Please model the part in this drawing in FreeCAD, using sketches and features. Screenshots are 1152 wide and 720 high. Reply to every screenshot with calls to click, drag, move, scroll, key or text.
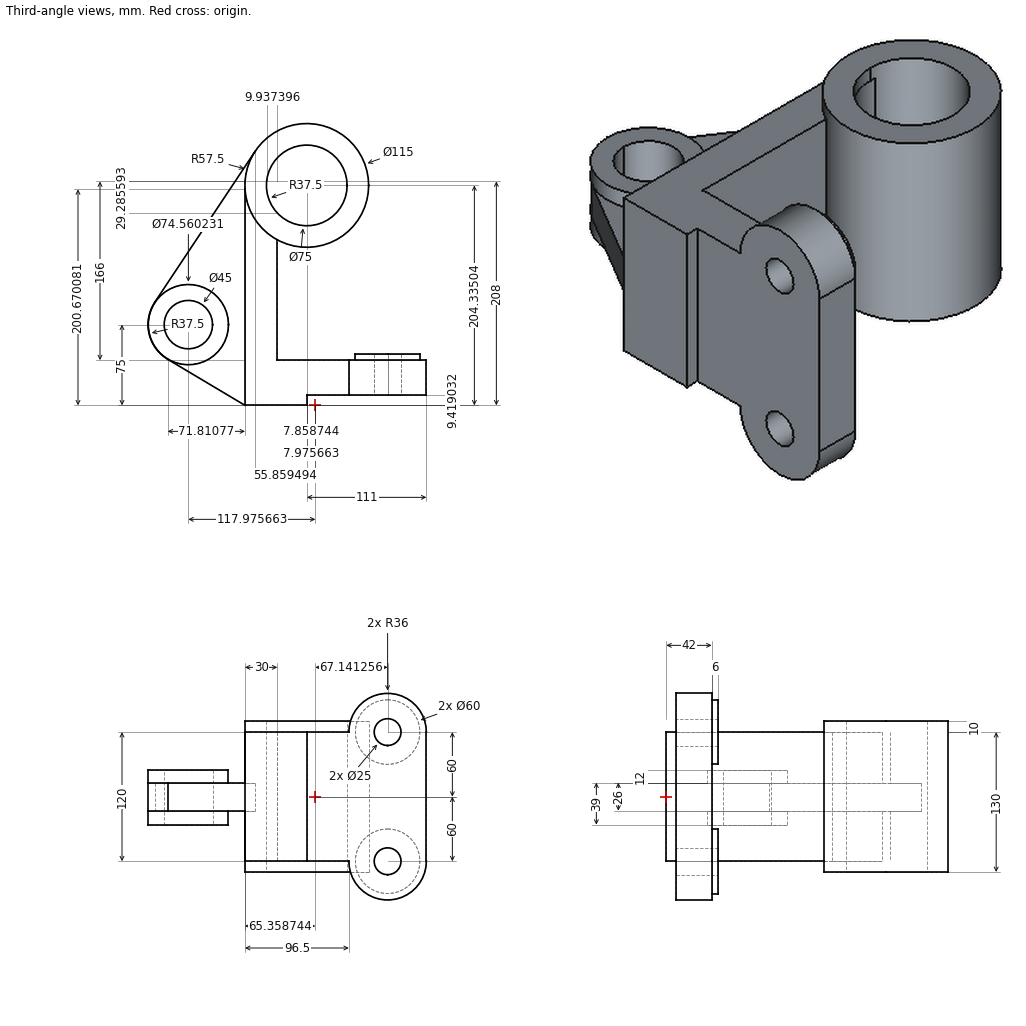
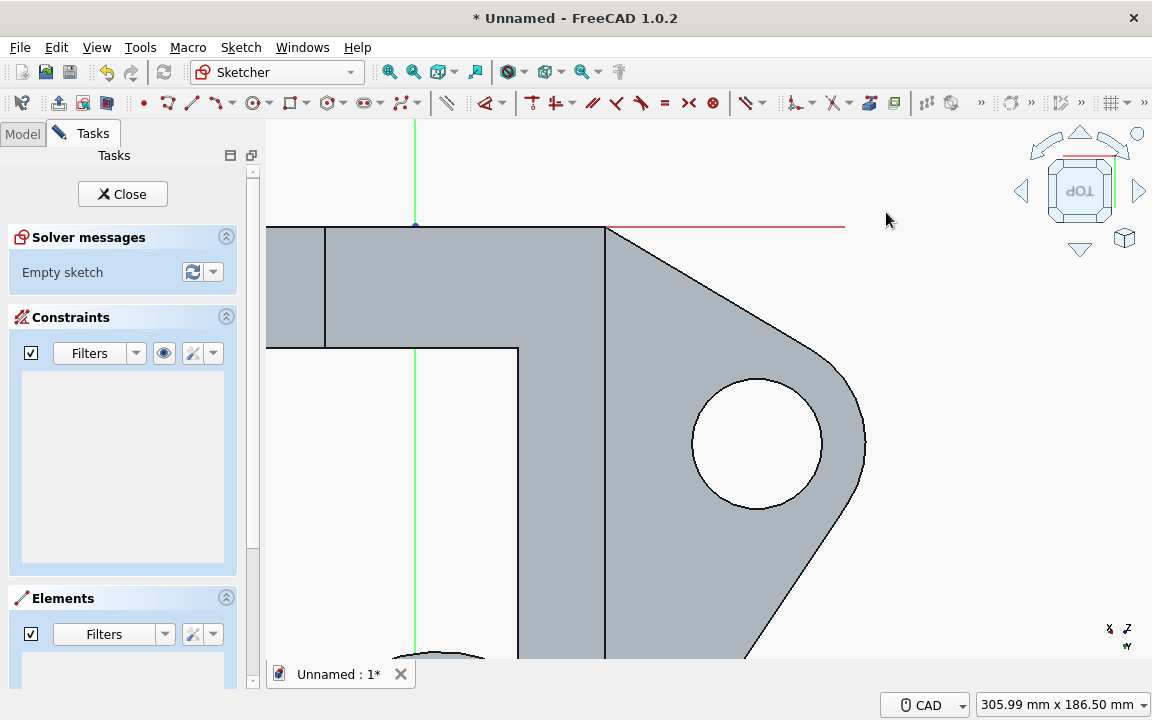
click(254, 104)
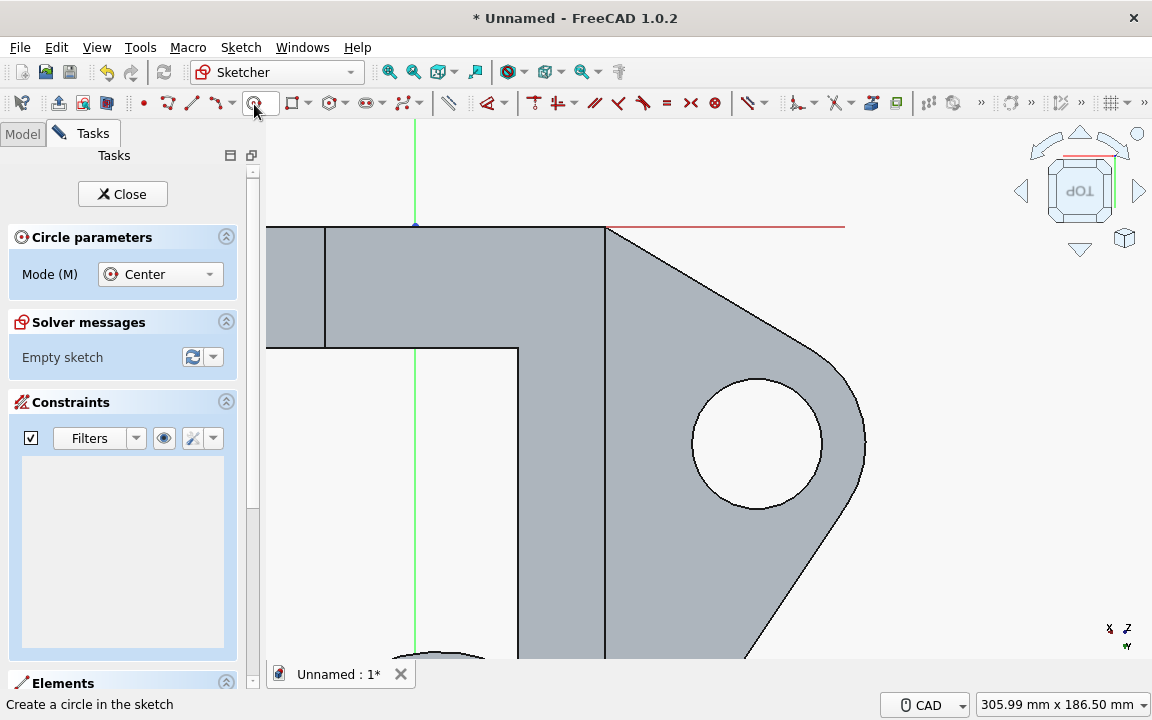
click(757, 444)
move(833, 368)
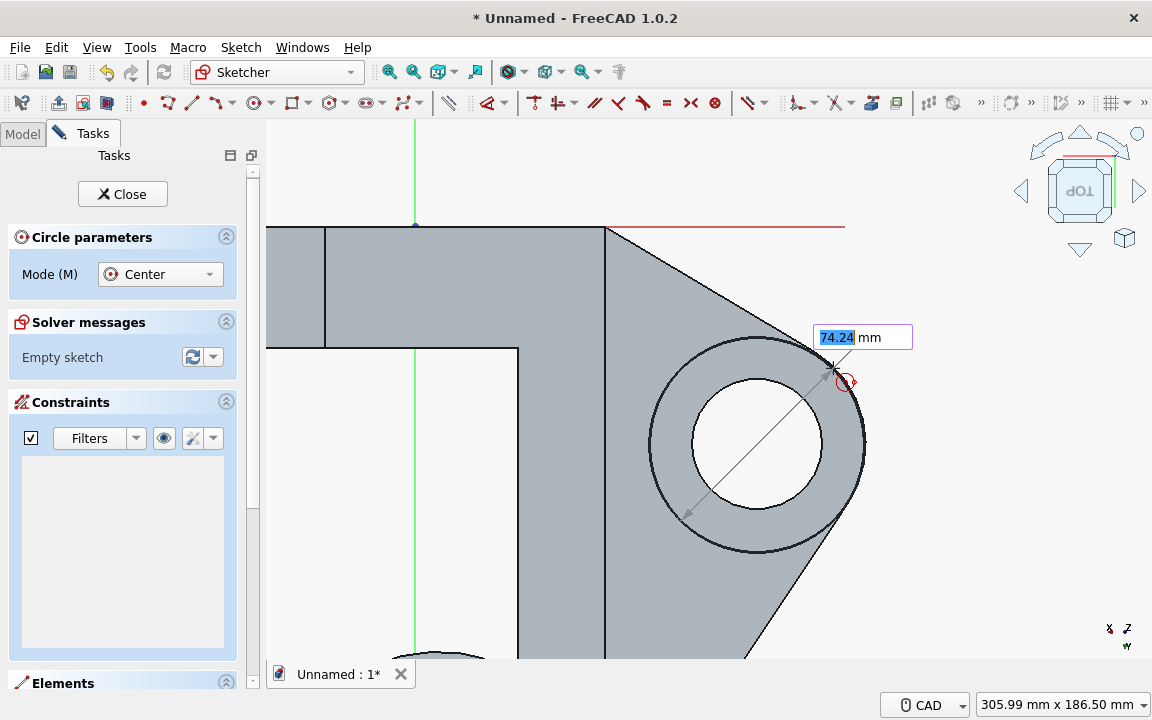
text(74.560231)
key(Return)
key(Escape)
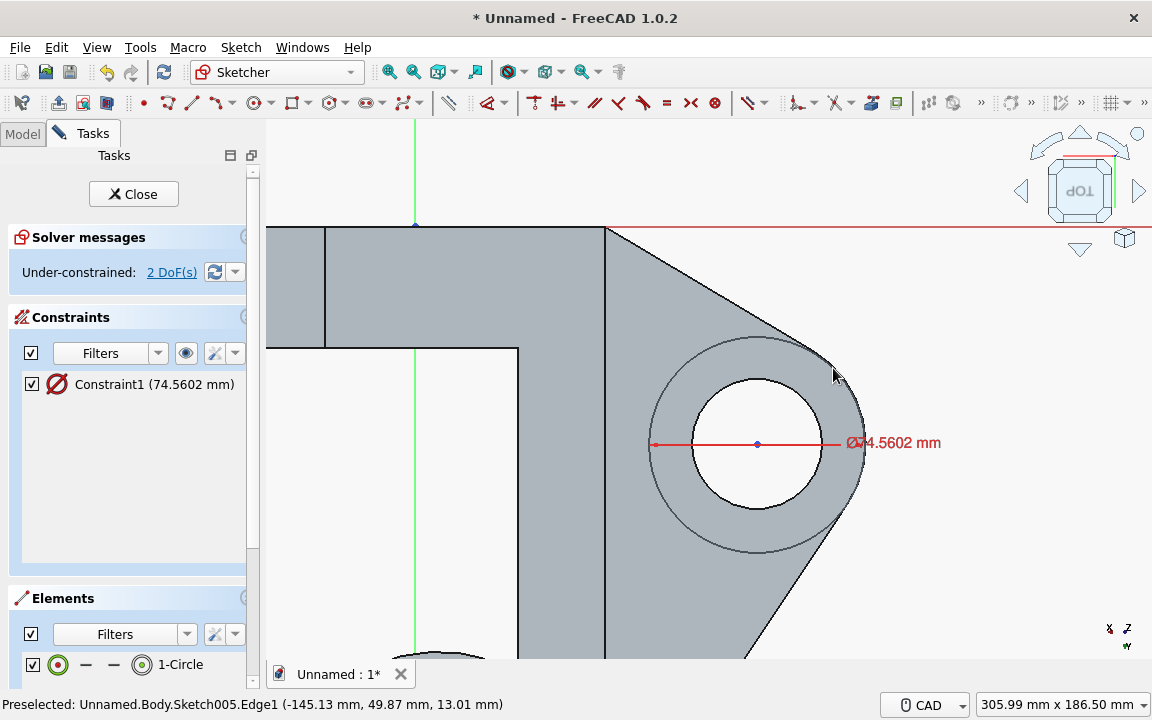
click(488, 104)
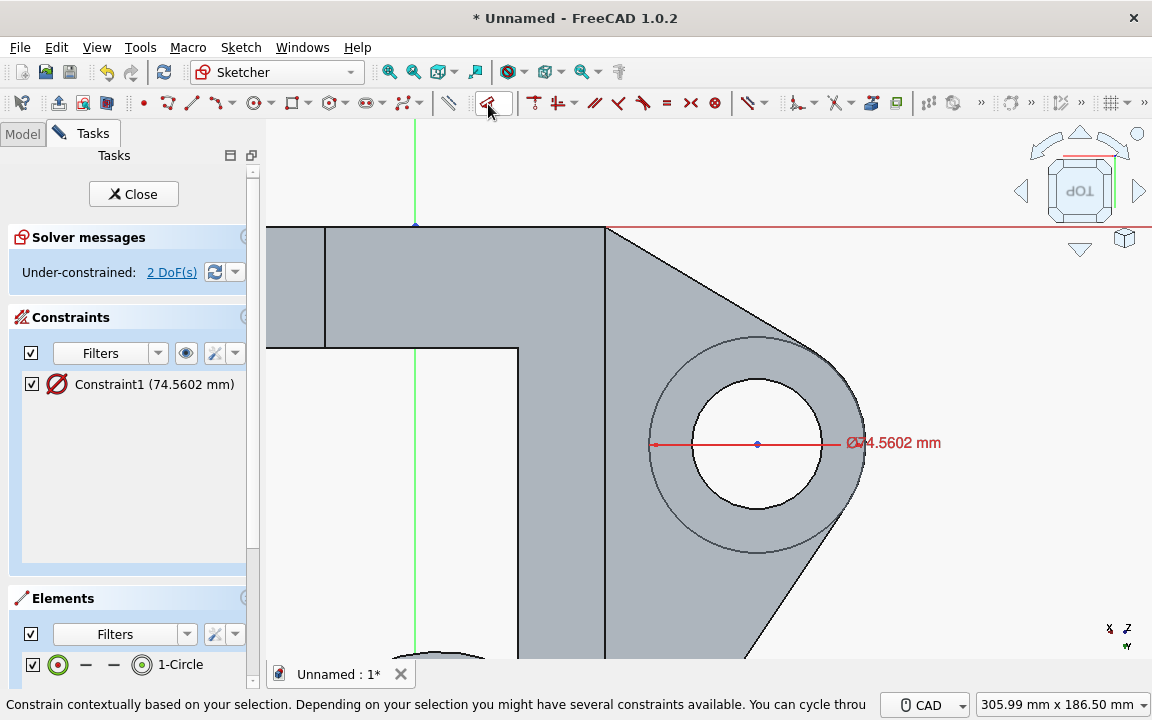
click(757, 445)
click(381, 336)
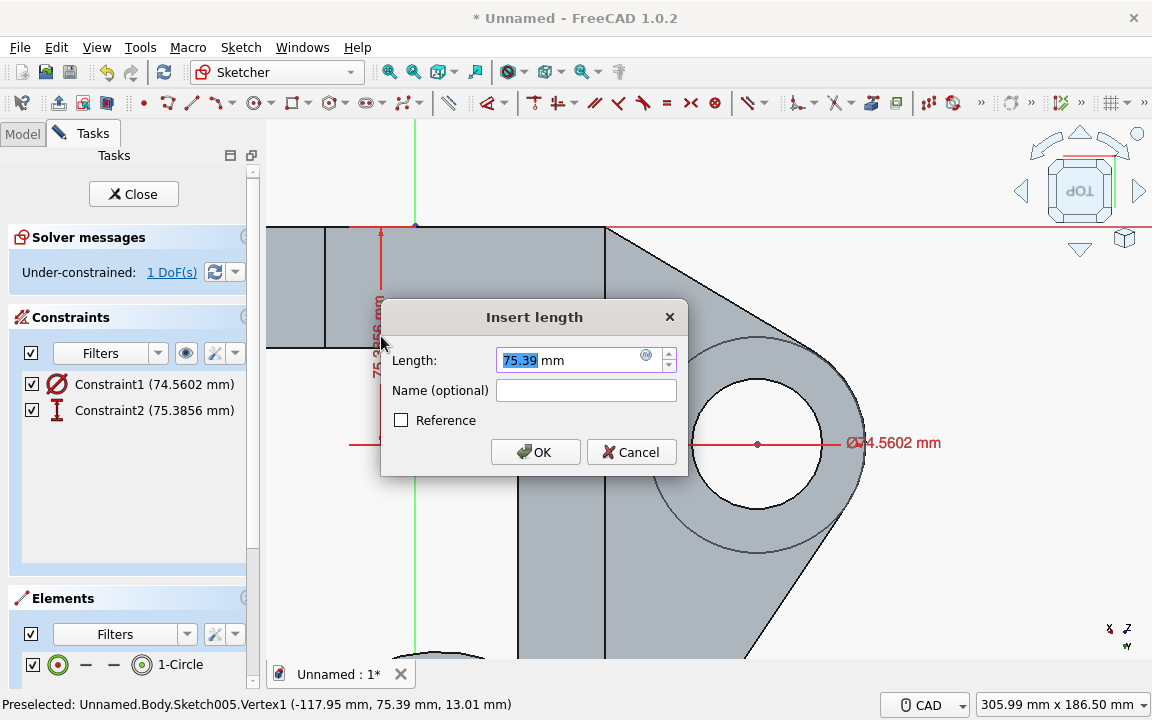
text(75)
key(Return)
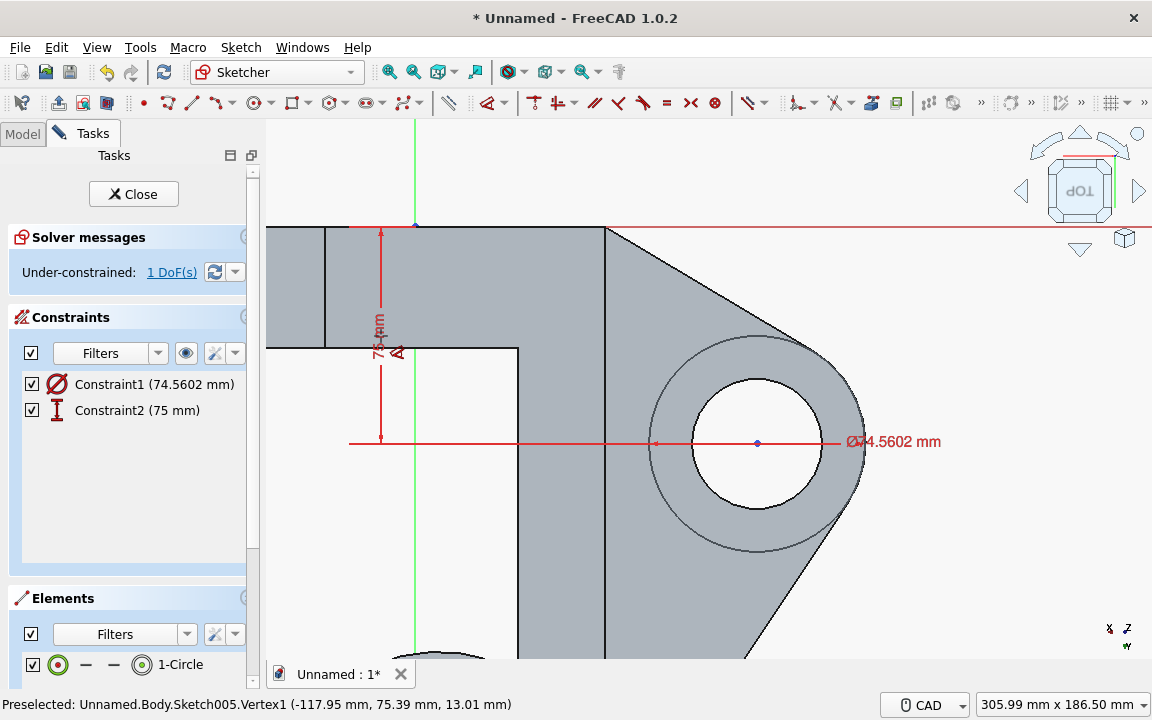
click(757, 444)
click(586, 193)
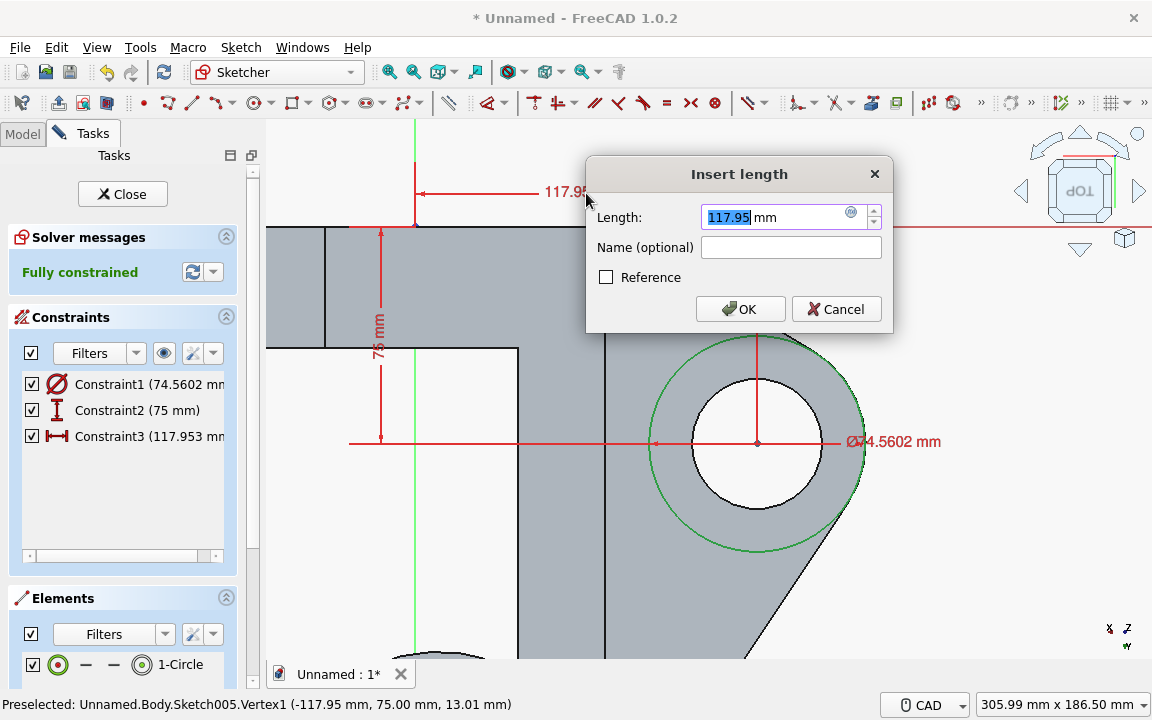
text(117.975663)
key(Return)
key(Escape)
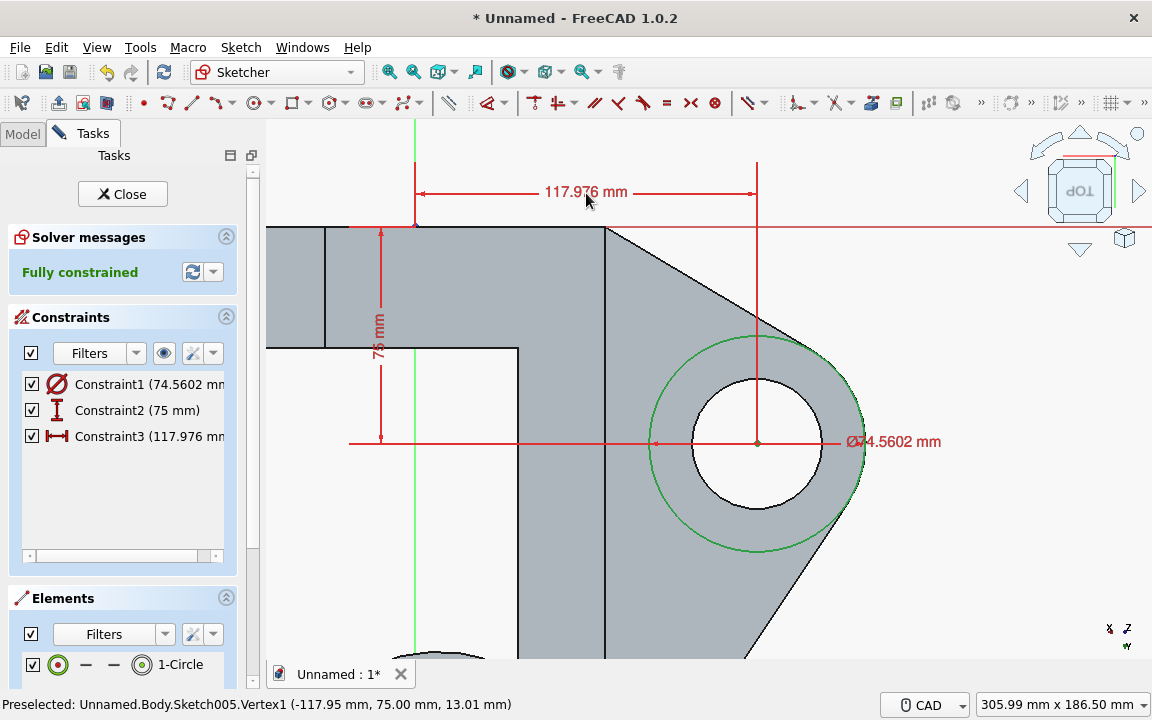
click(123, 194)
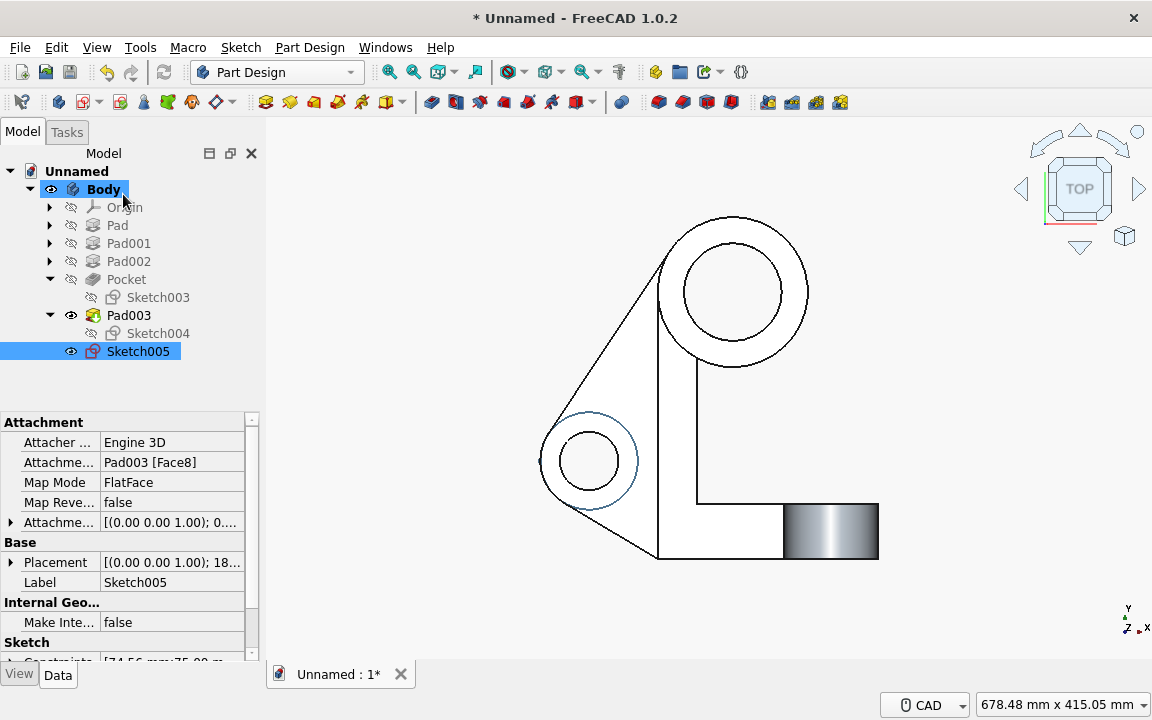
click(266, 102)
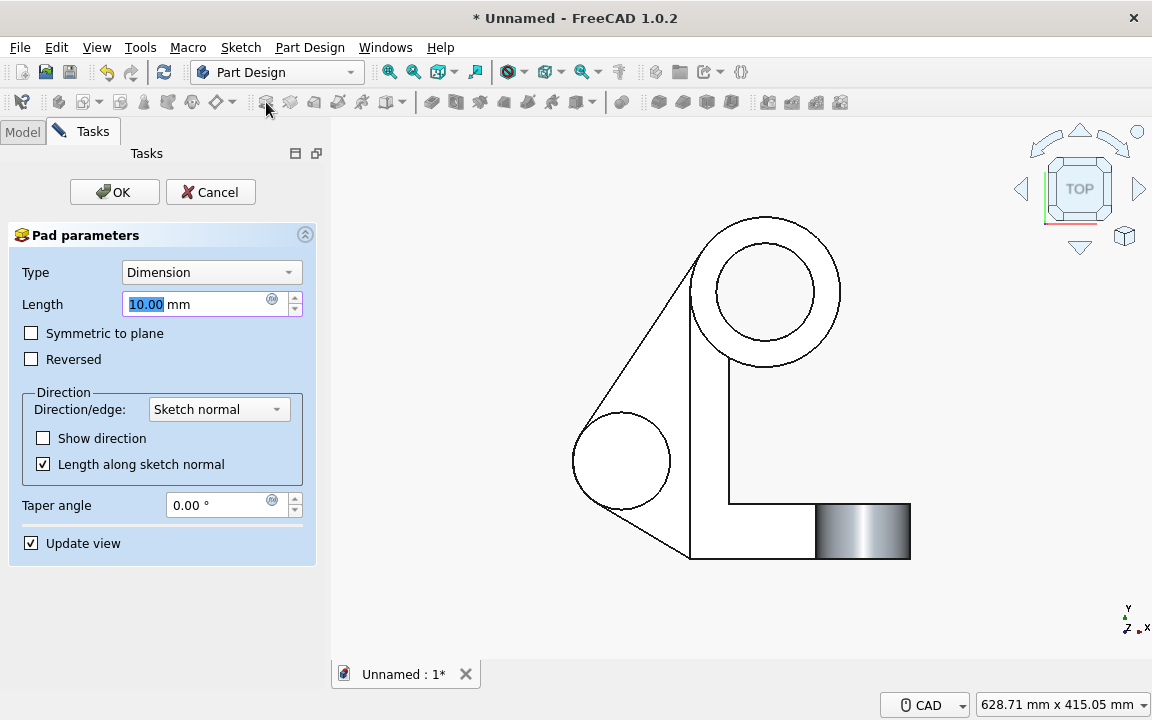
click(212, 272)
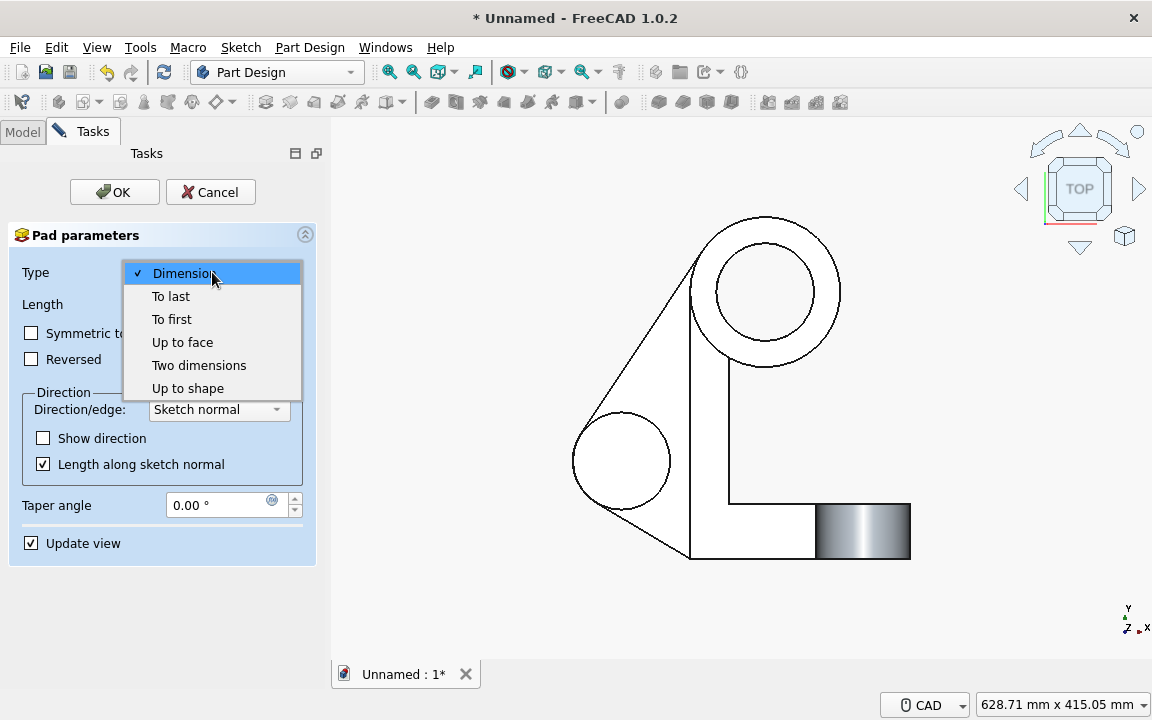
click(212, 366)